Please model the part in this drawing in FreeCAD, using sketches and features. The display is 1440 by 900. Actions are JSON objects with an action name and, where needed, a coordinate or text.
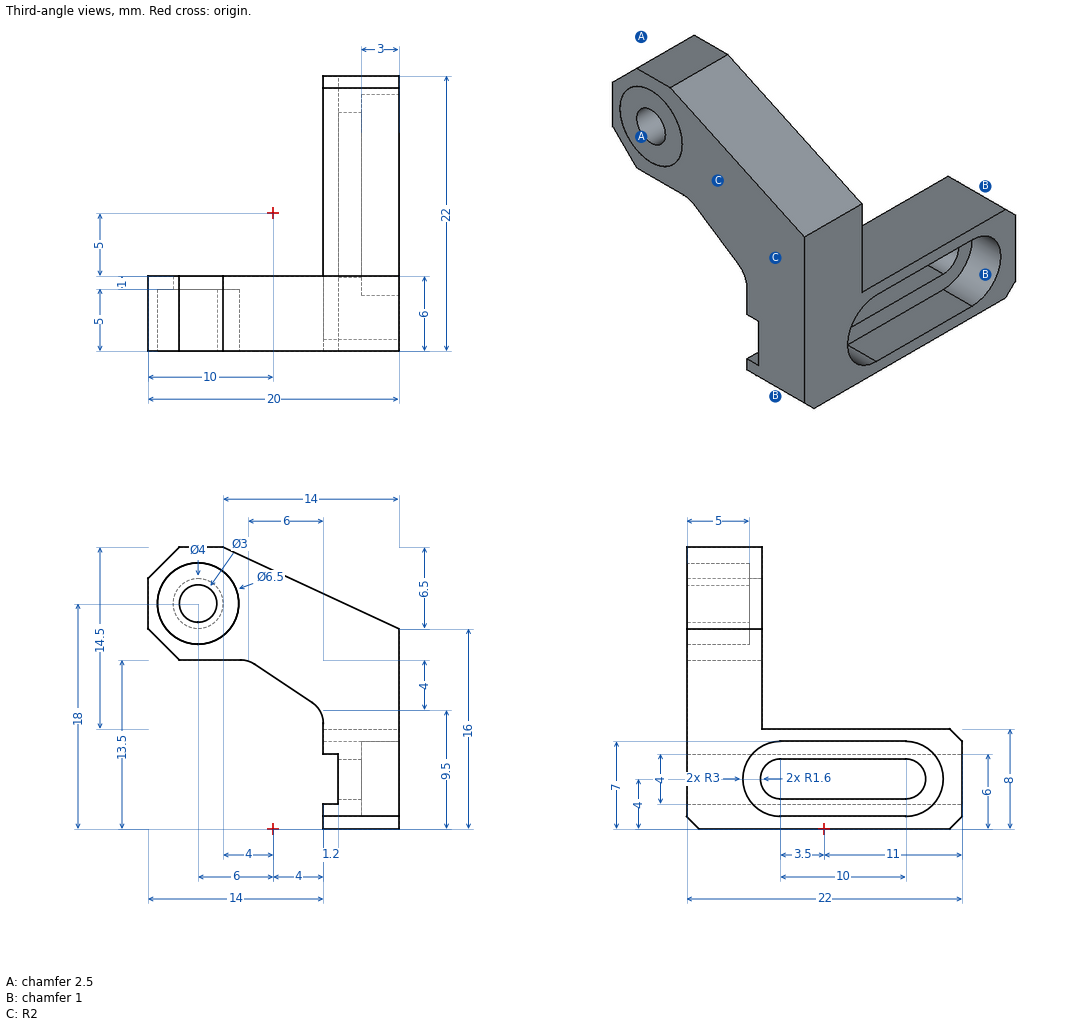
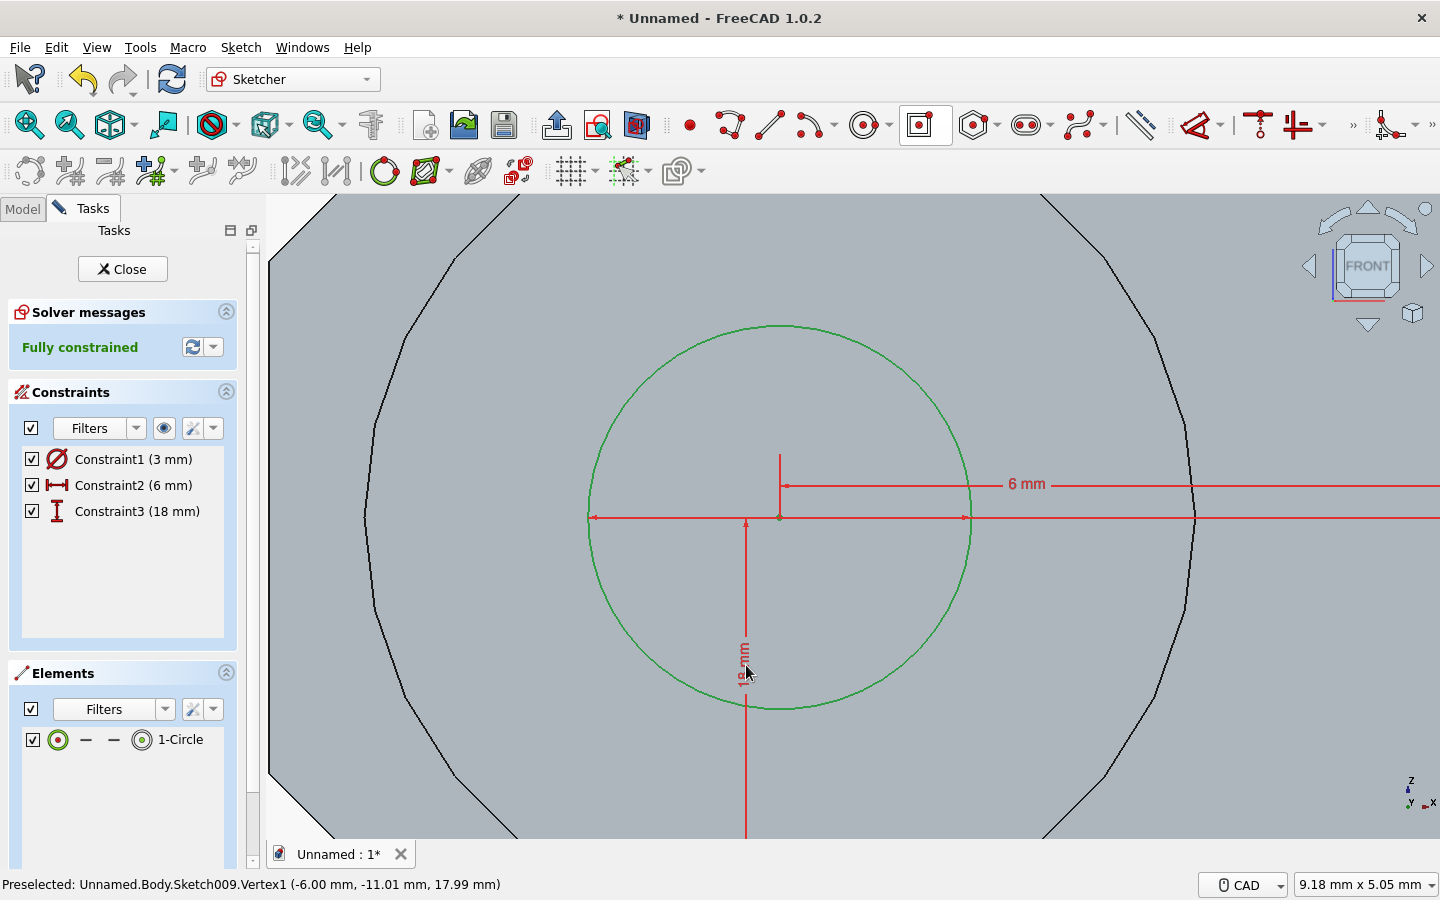
{"action": "left_click", "coordinate": [123, 269]}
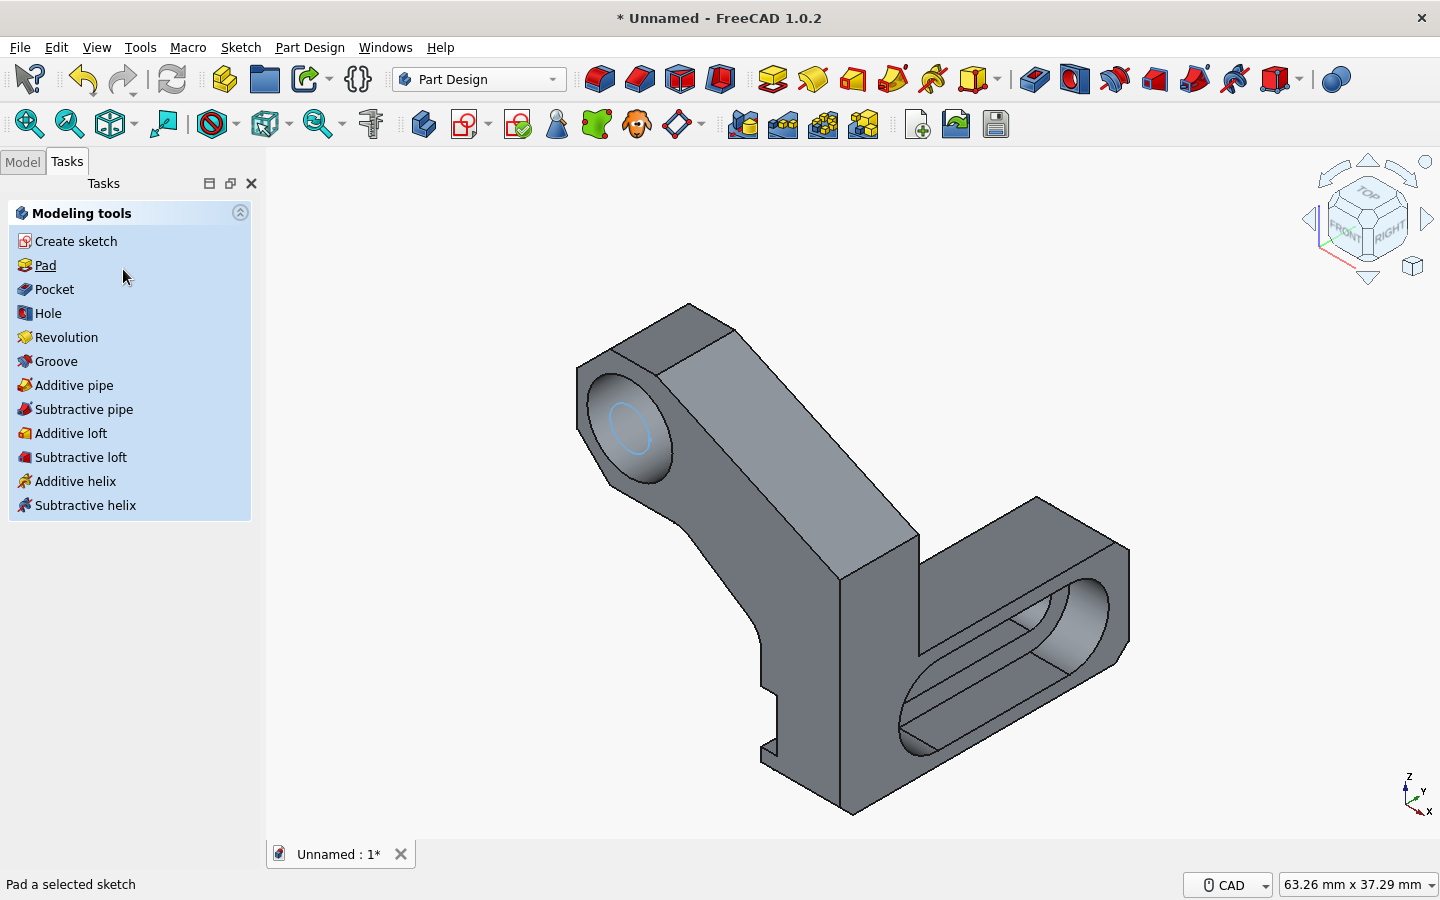
{"action": "left_click", "coordinate": [1036, 80]}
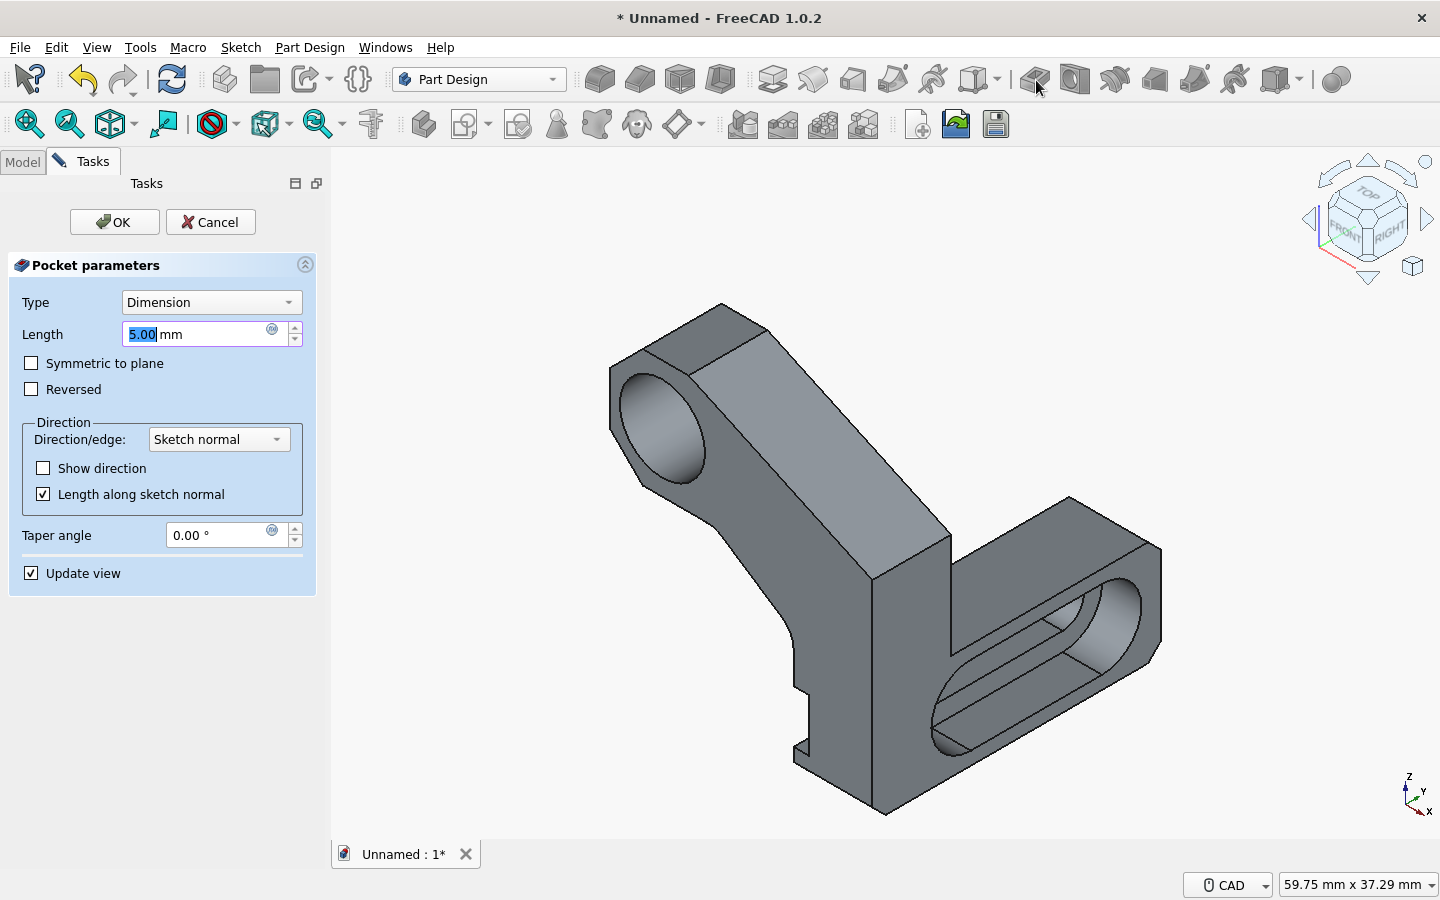
{"action": "left_click", "coordinate": [212, 302]}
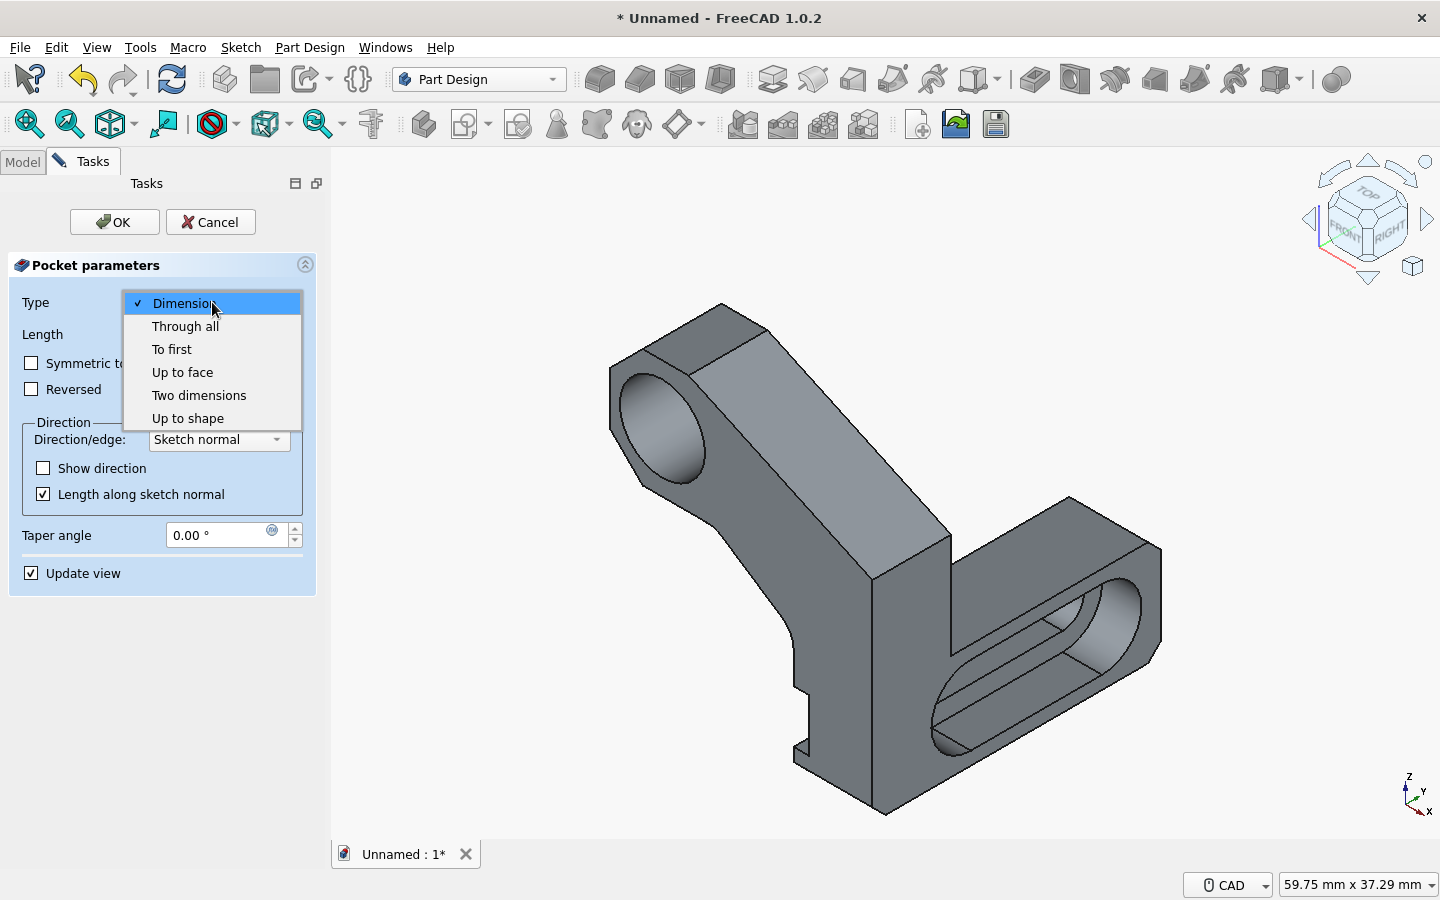
{"action": "left_click", "coordinate": [212, 326]}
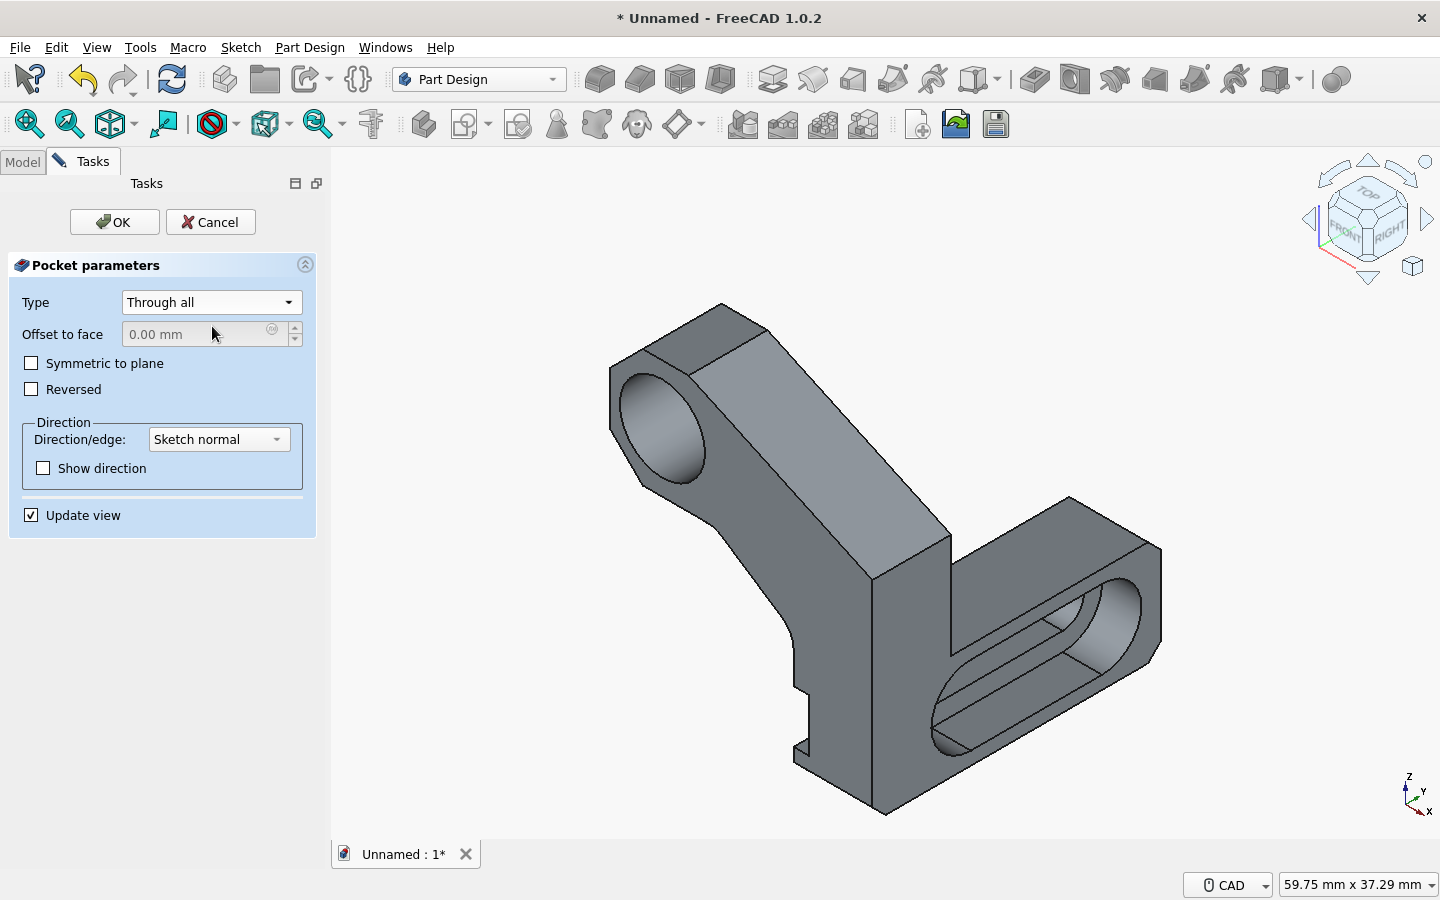
{"action": "left_click", "coordinate": [115, 222]}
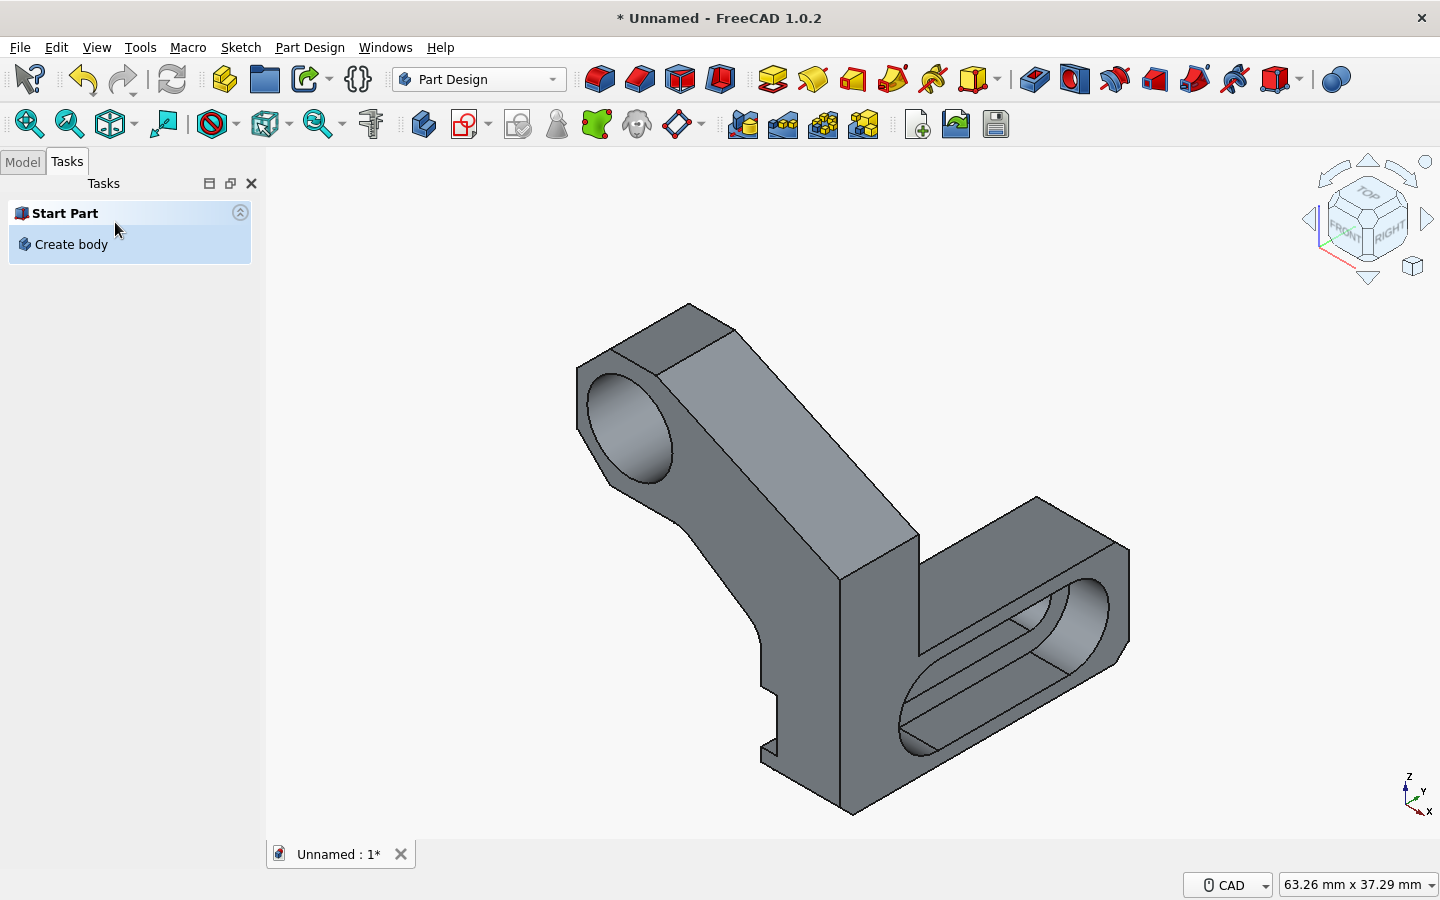
{"action": "key", "text": "4"}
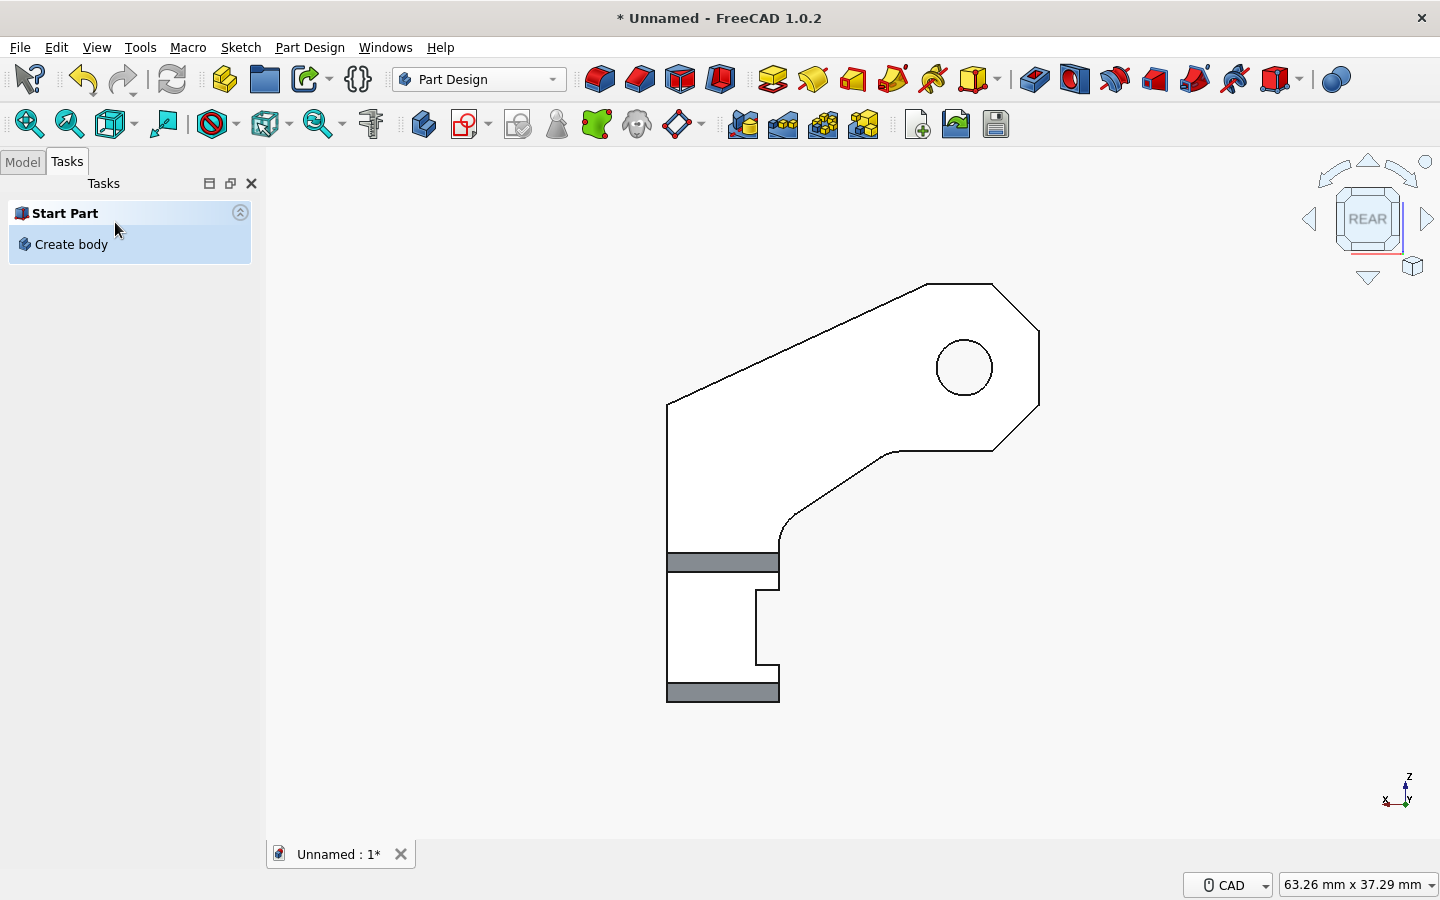
{"action": "left_click", "coordinate": [747, 456]}